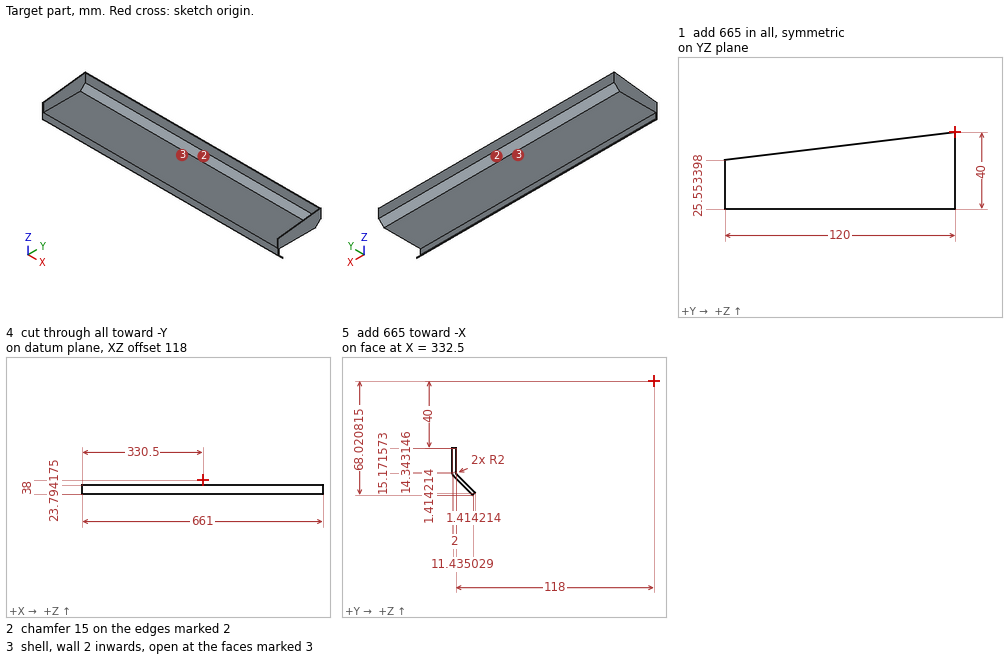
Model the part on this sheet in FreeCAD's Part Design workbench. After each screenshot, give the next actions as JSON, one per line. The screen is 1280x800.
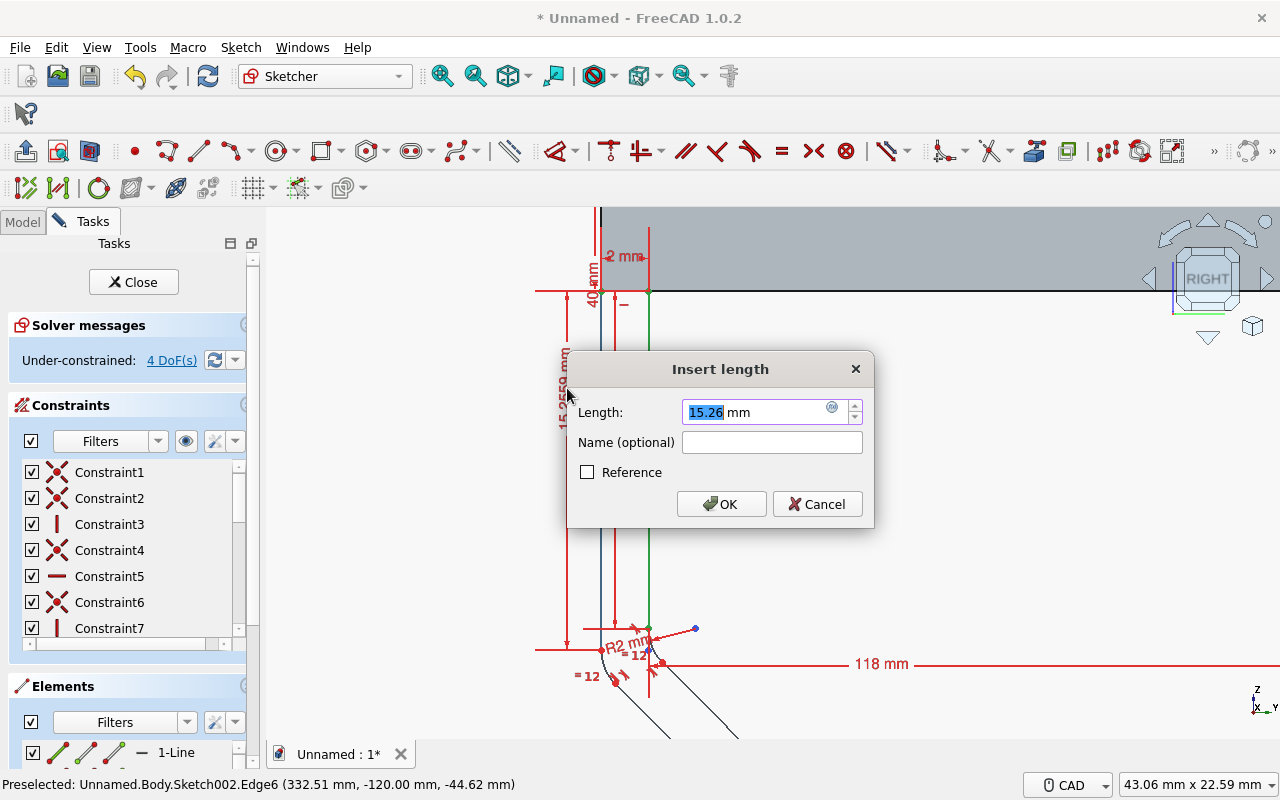
{"action": "type", "text": "15.171573"}
{"action": "key", "text": "Return"}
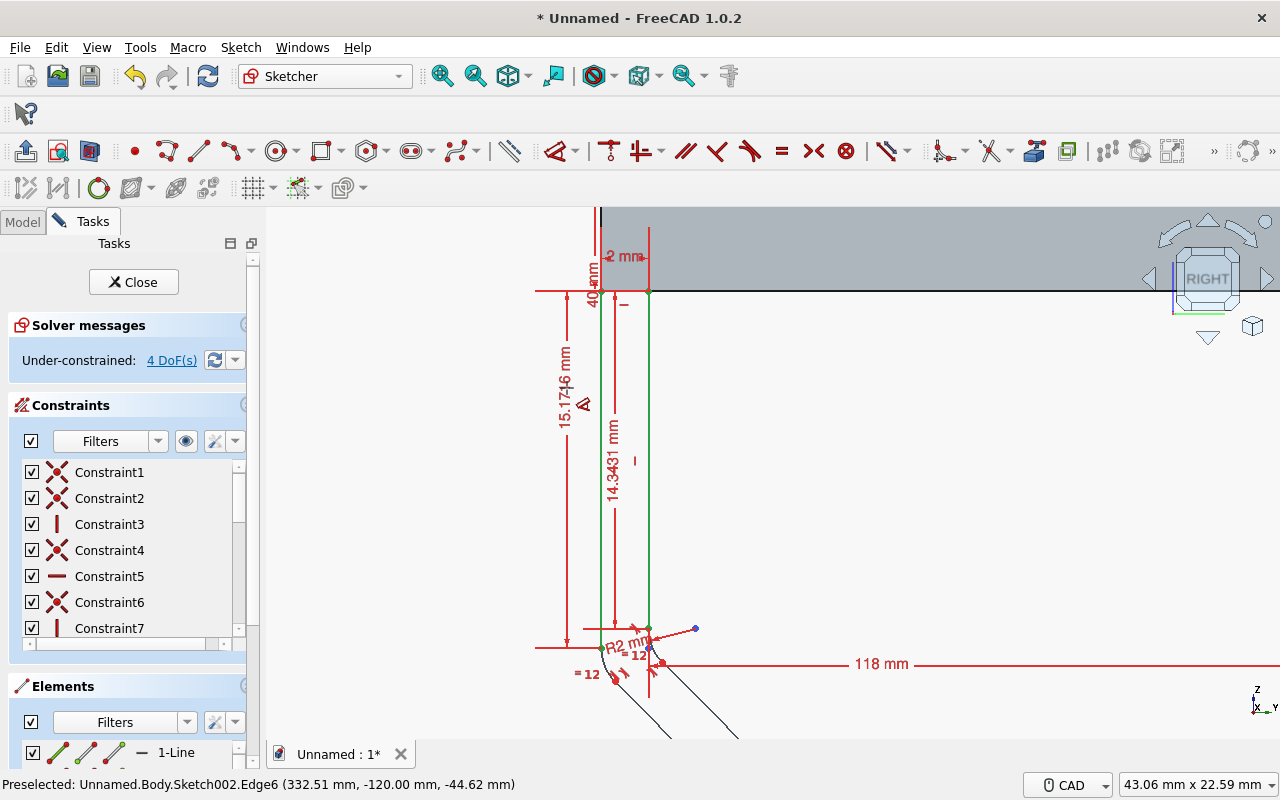
{"action": "scroll", "coordinate": [637, 293], "scroll_direction": "down", "scroll_amount": 3}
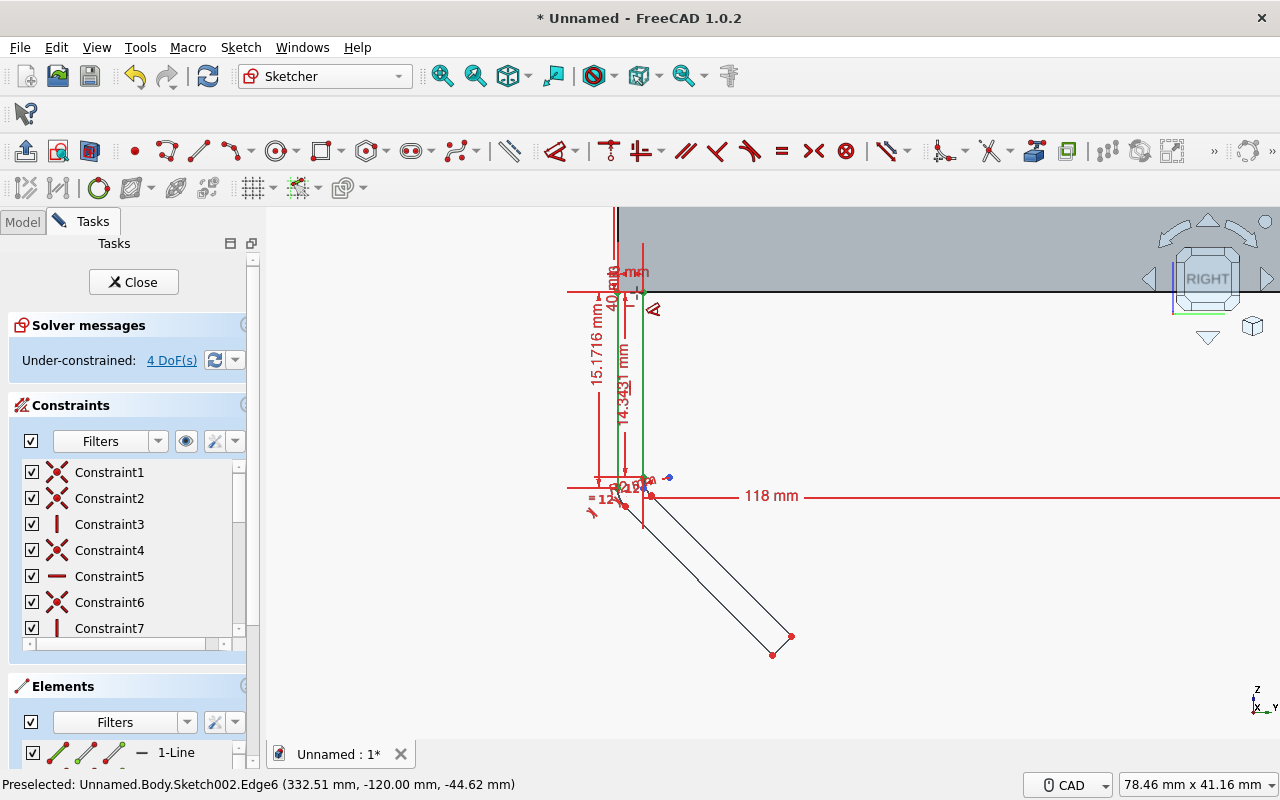
{"action": "scroll", "coordinate": [778, 650], "scroll_direction": "up", "scroll_amount": 4}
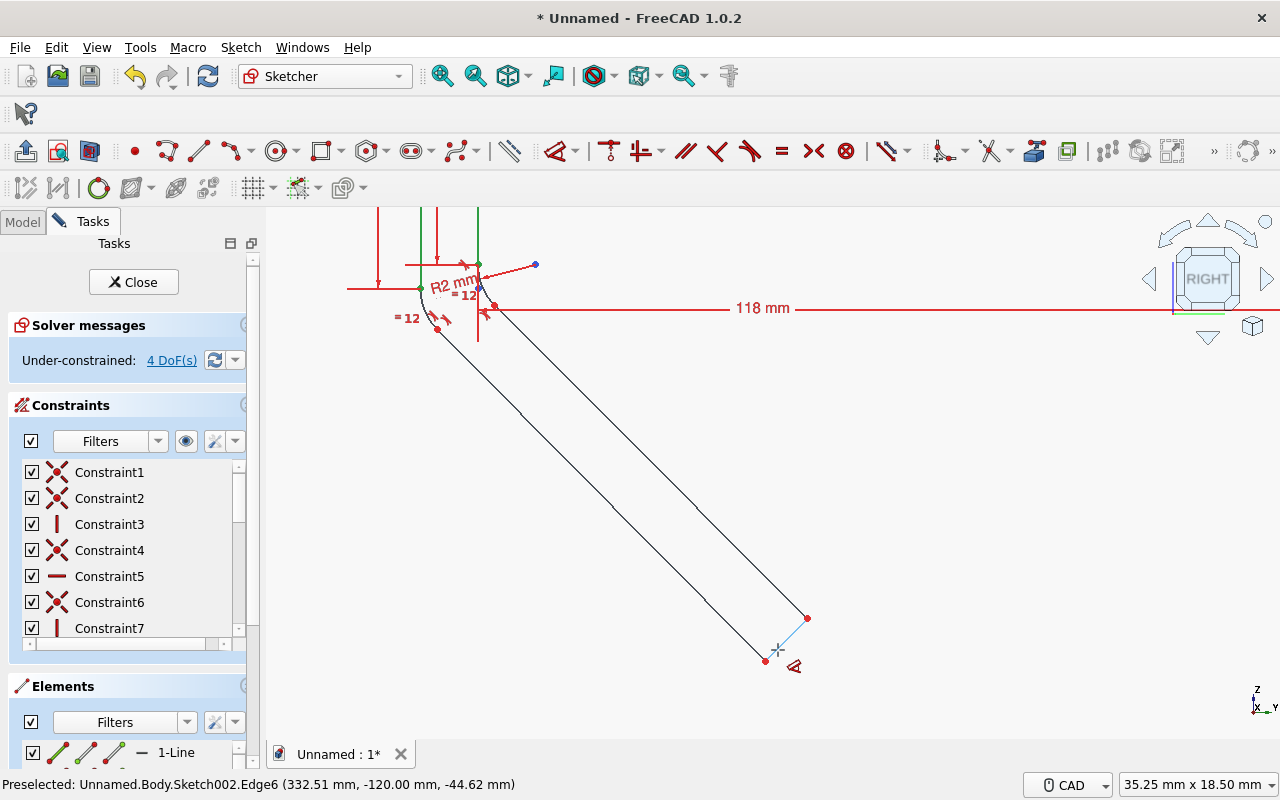
{"action": "left_click", "coordinate": [778, 649]}
{"action": "left_click", "coordinate": [787, 695]}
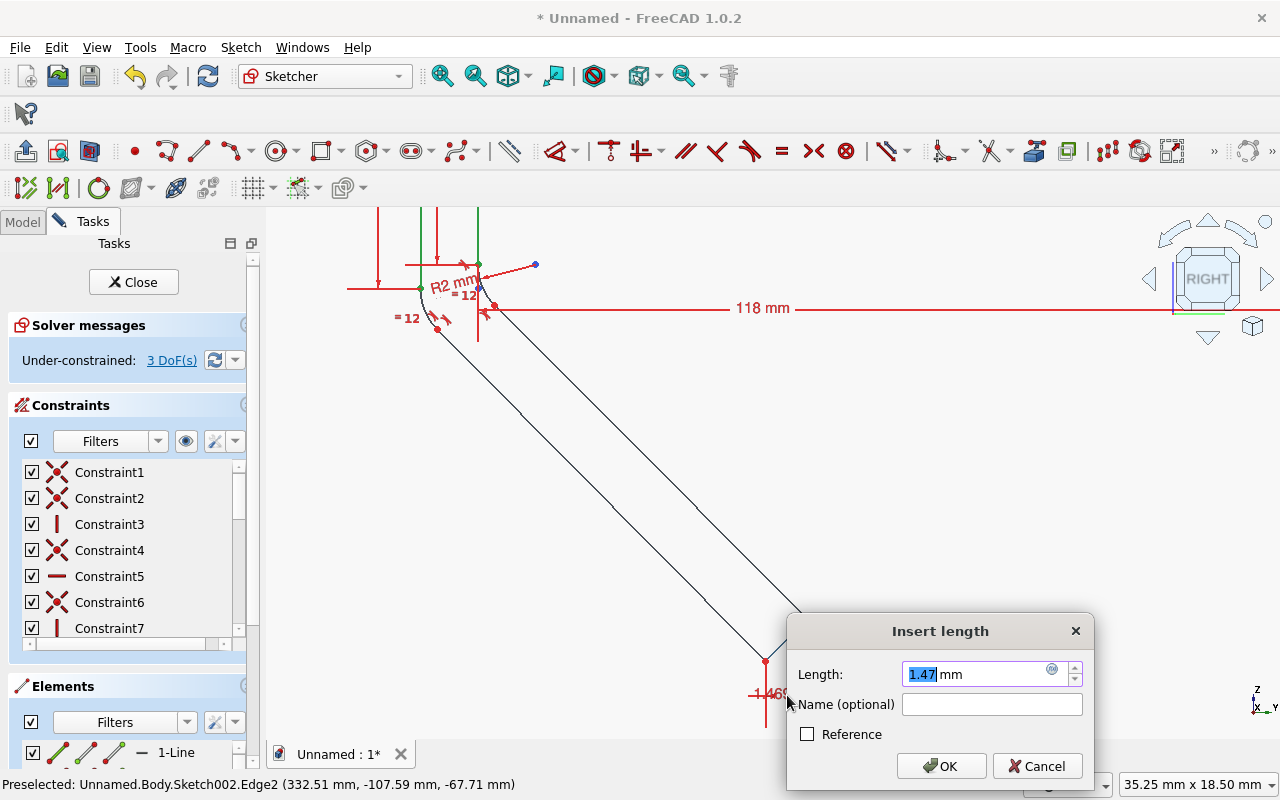
{"action": "type", "text": "1.414214"}
{"action": "key", "text": "Return"}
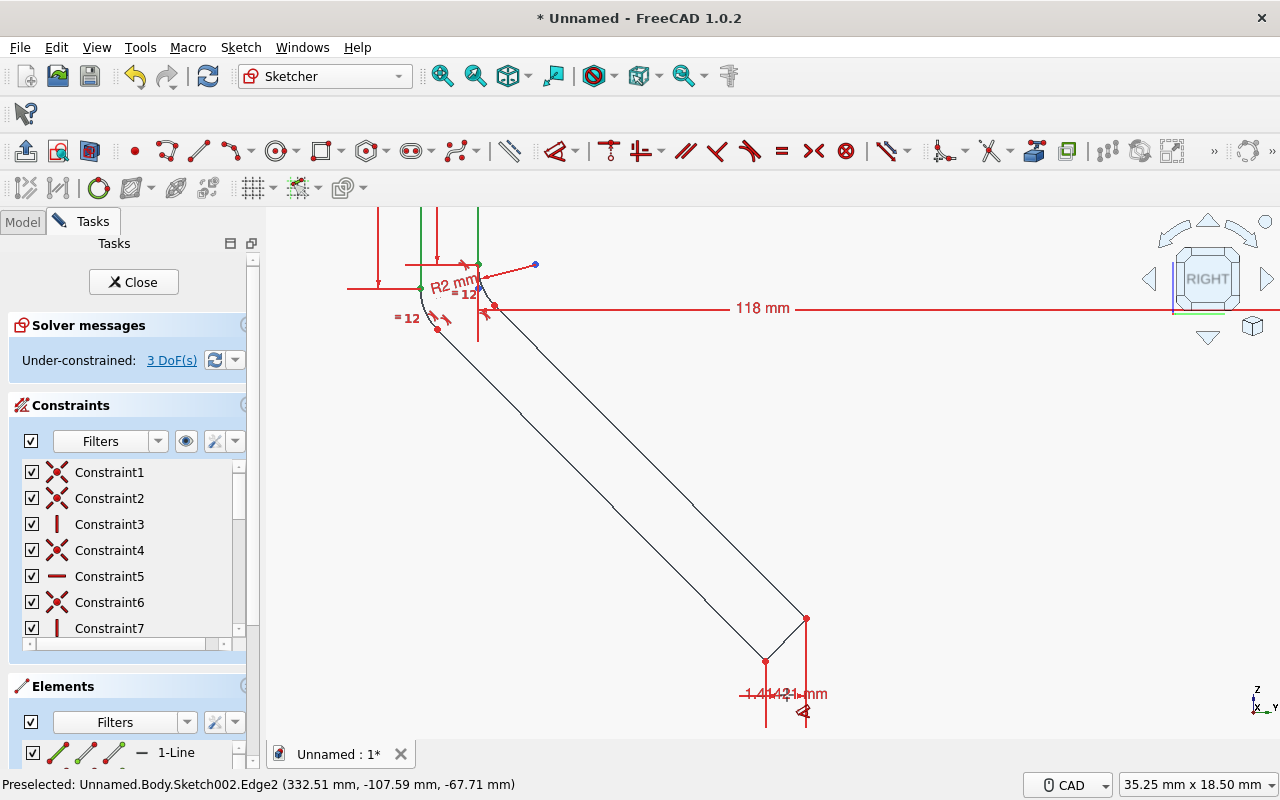
{"action": "left_click", "coordinate": [778, 649]}
{"action": "left_click", "coordinate": [840, 640]}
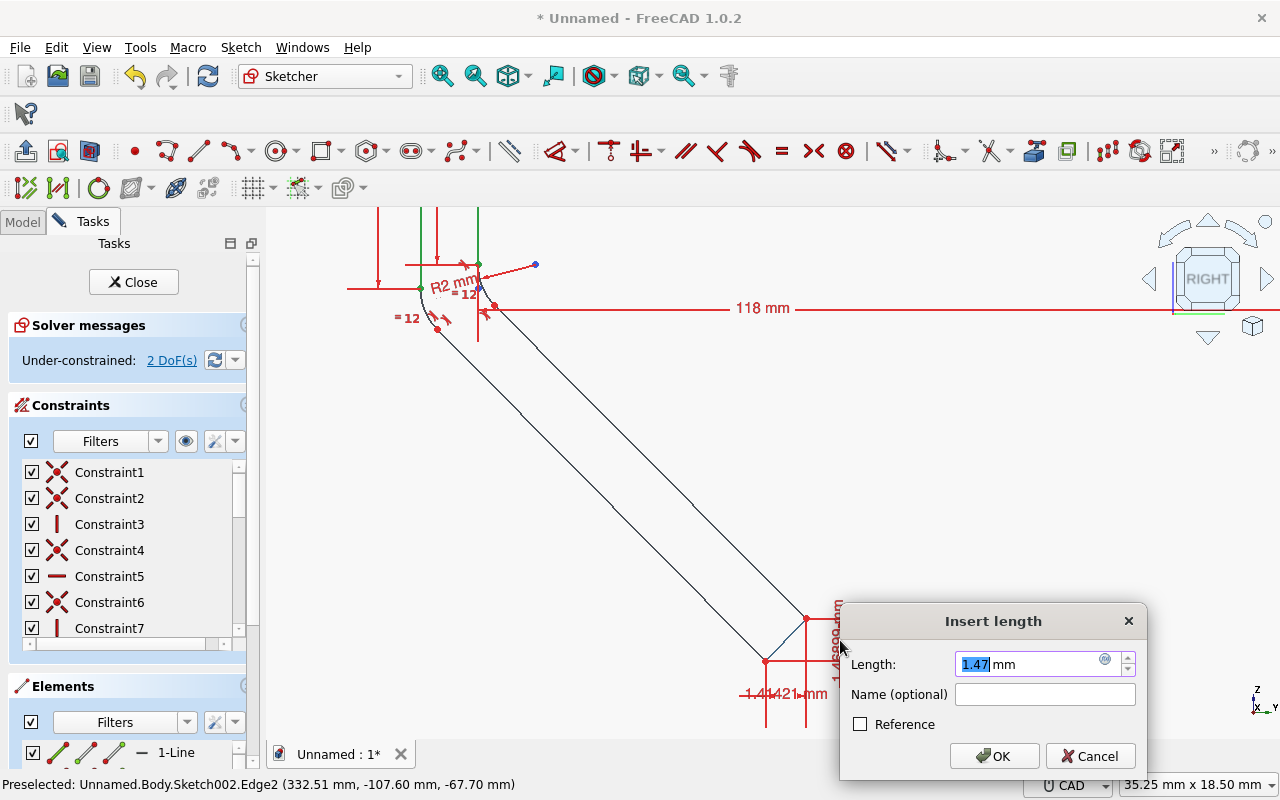
{"action": "type", "text": "1.414214"}
{"action": "key", "text": "Return"}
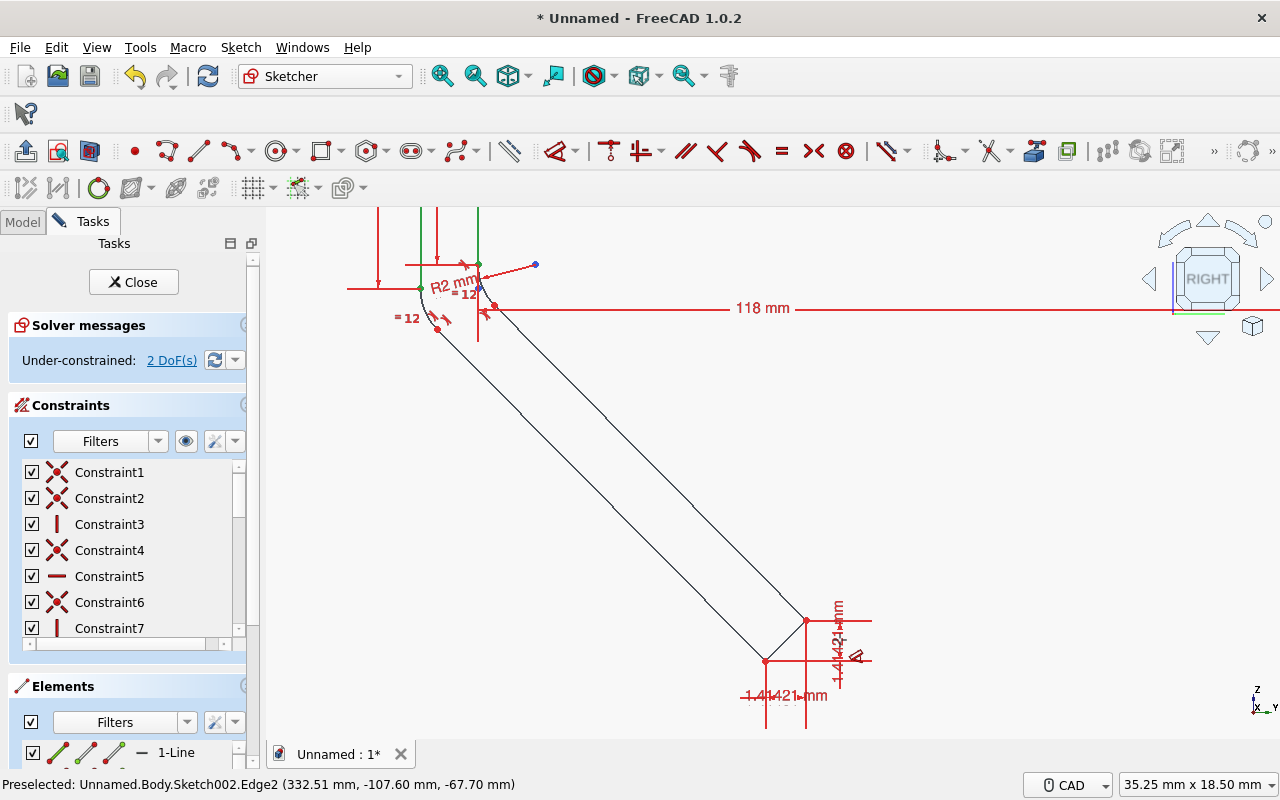
{"action": "left_click", "coordinate": [766, 661]}
{"action": "left_click", "coordinate": [732, 448]}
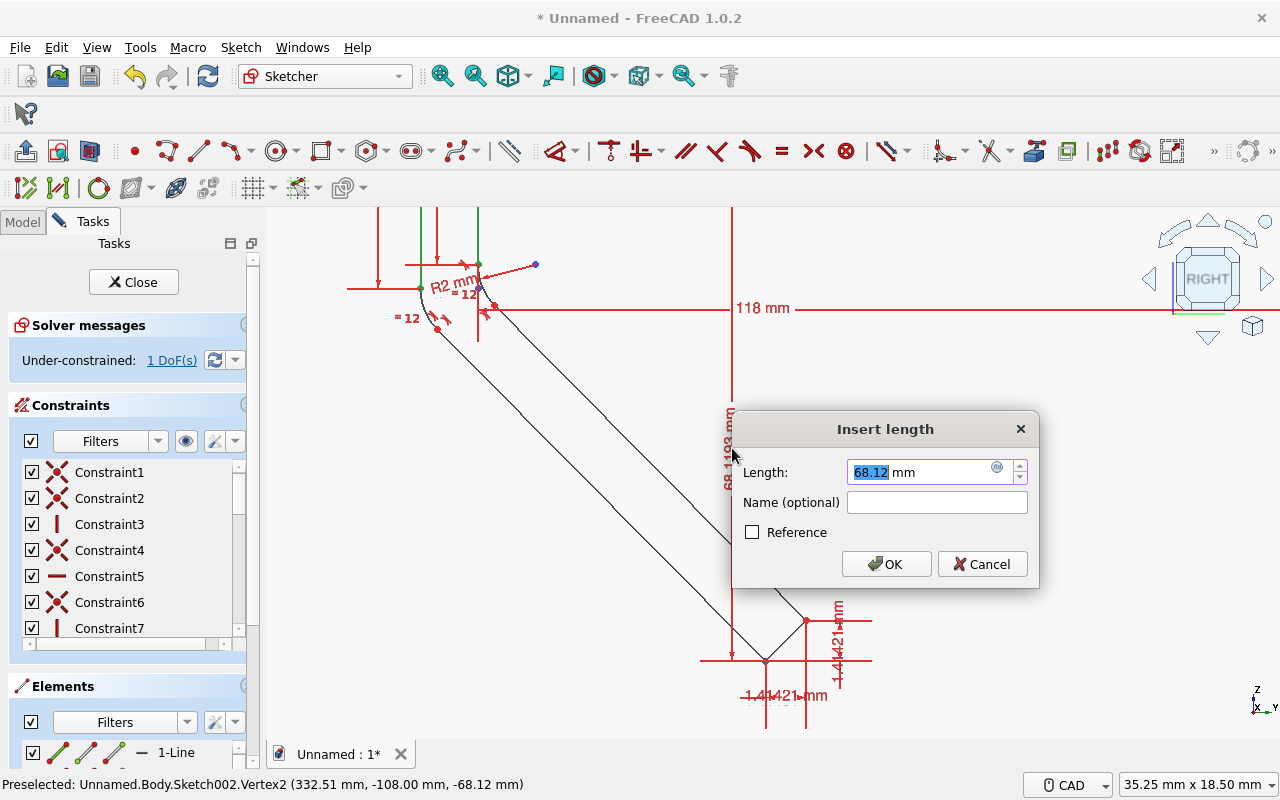
{"action": "type", "text": "68.020815"}
{"action": "key", "text": "Return"}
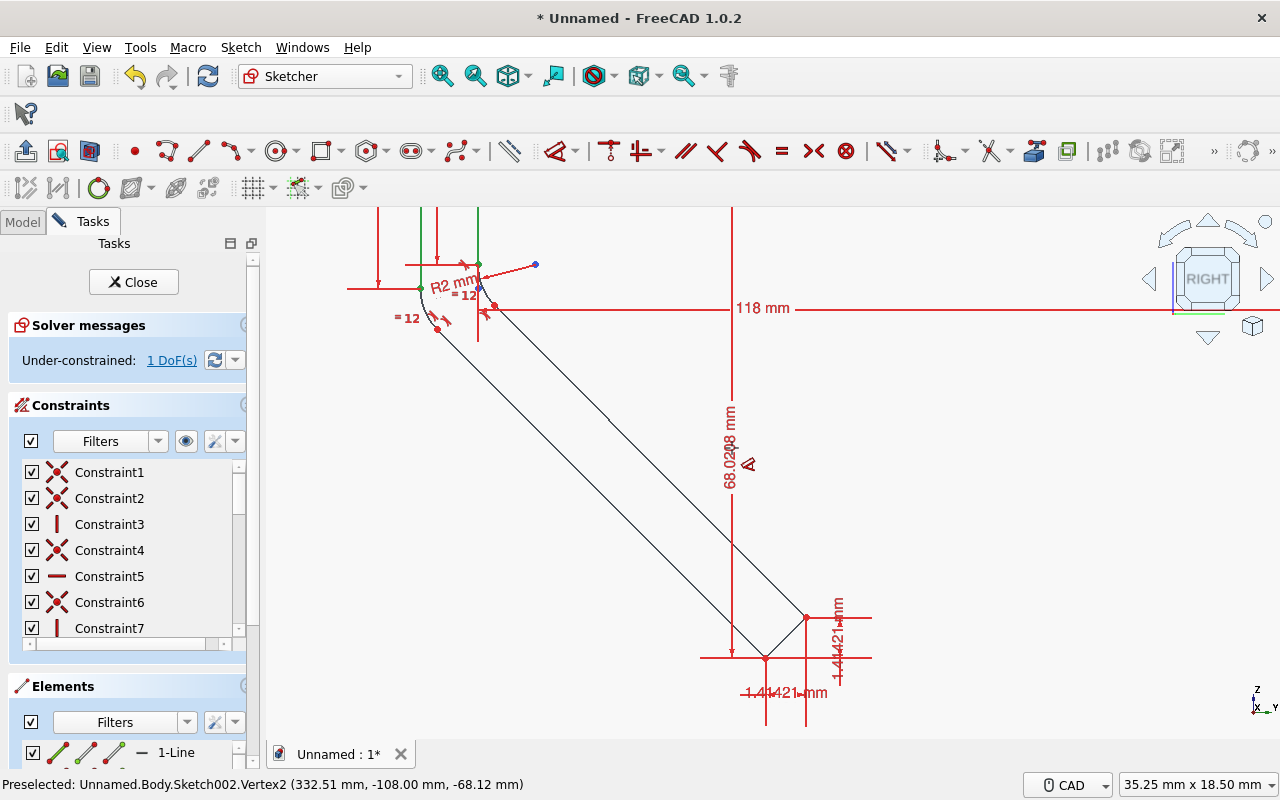
{"action": "left_click", "coordinate": [536, 428]}
{"action": "left_click", "coordinate": [601, 692]}